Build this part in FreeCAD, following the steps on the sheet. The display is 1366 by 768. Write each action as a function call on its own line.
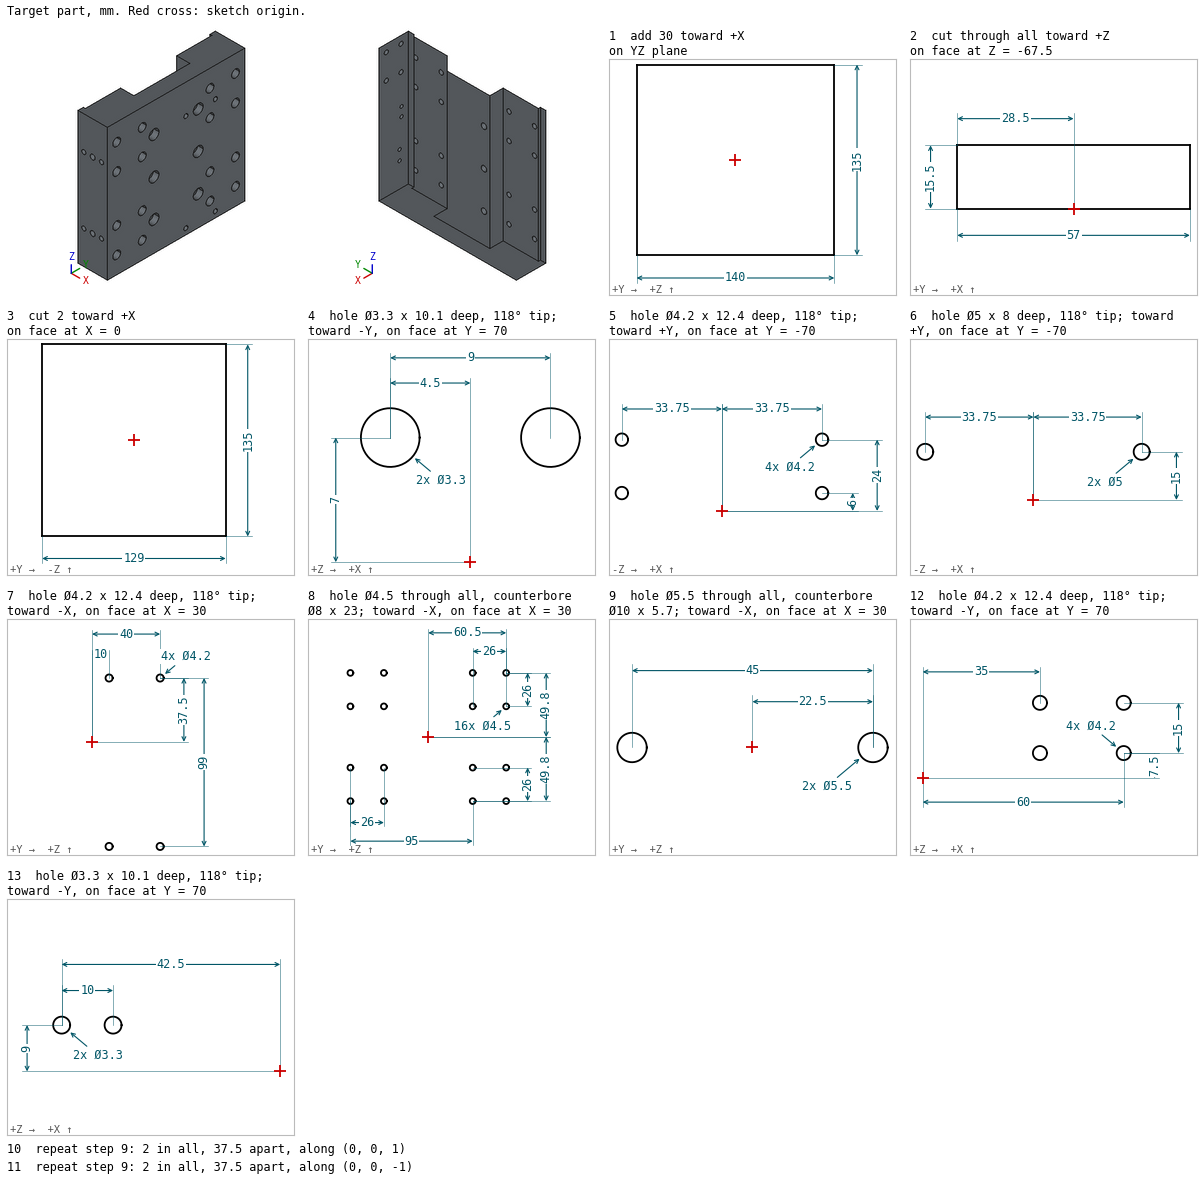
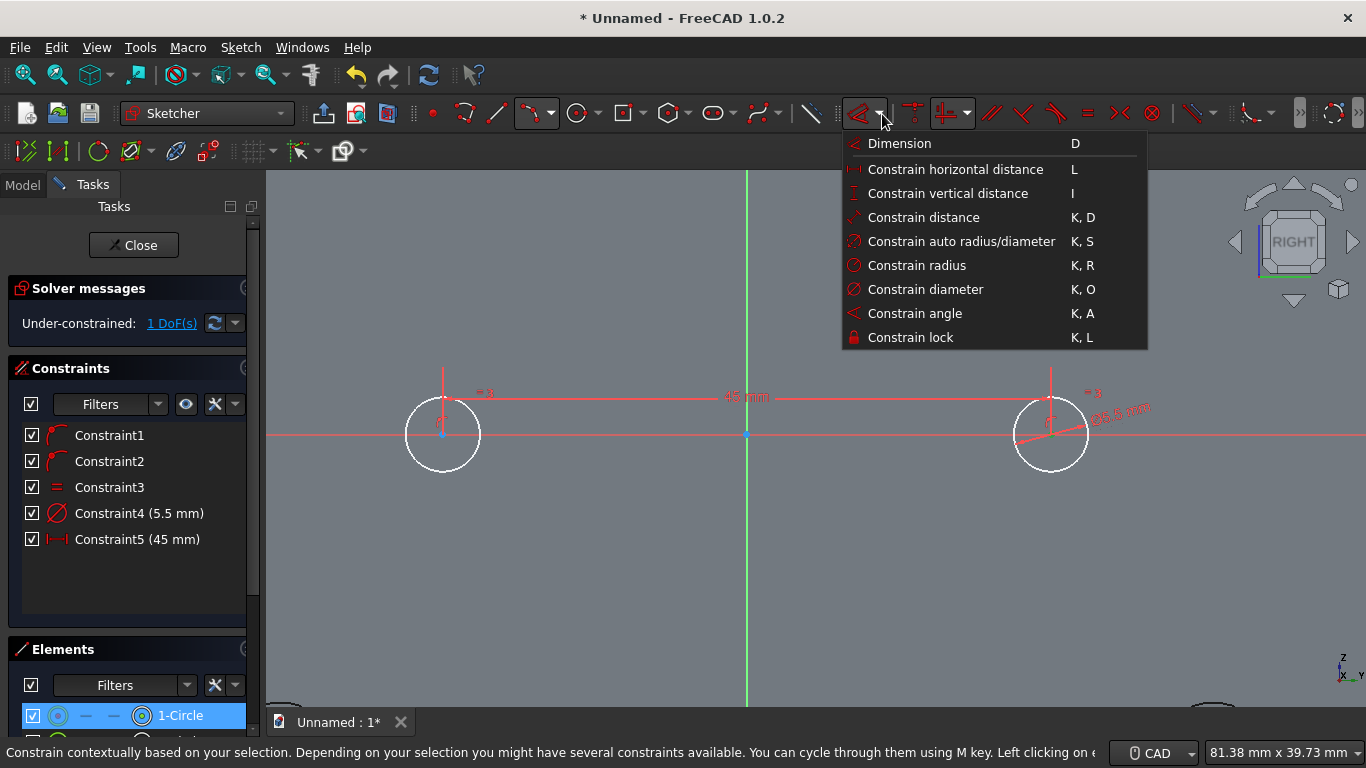
click(995, 169)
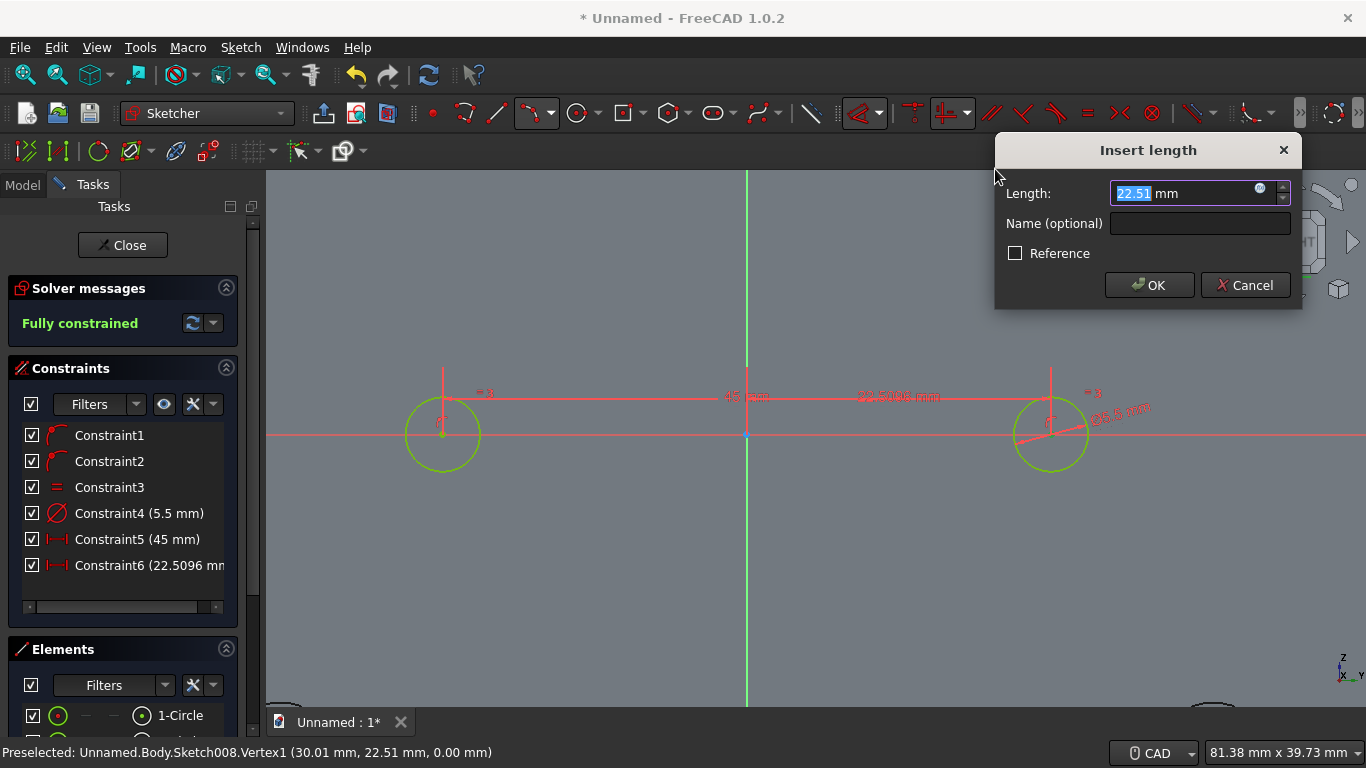
text(22.5)
key(Return)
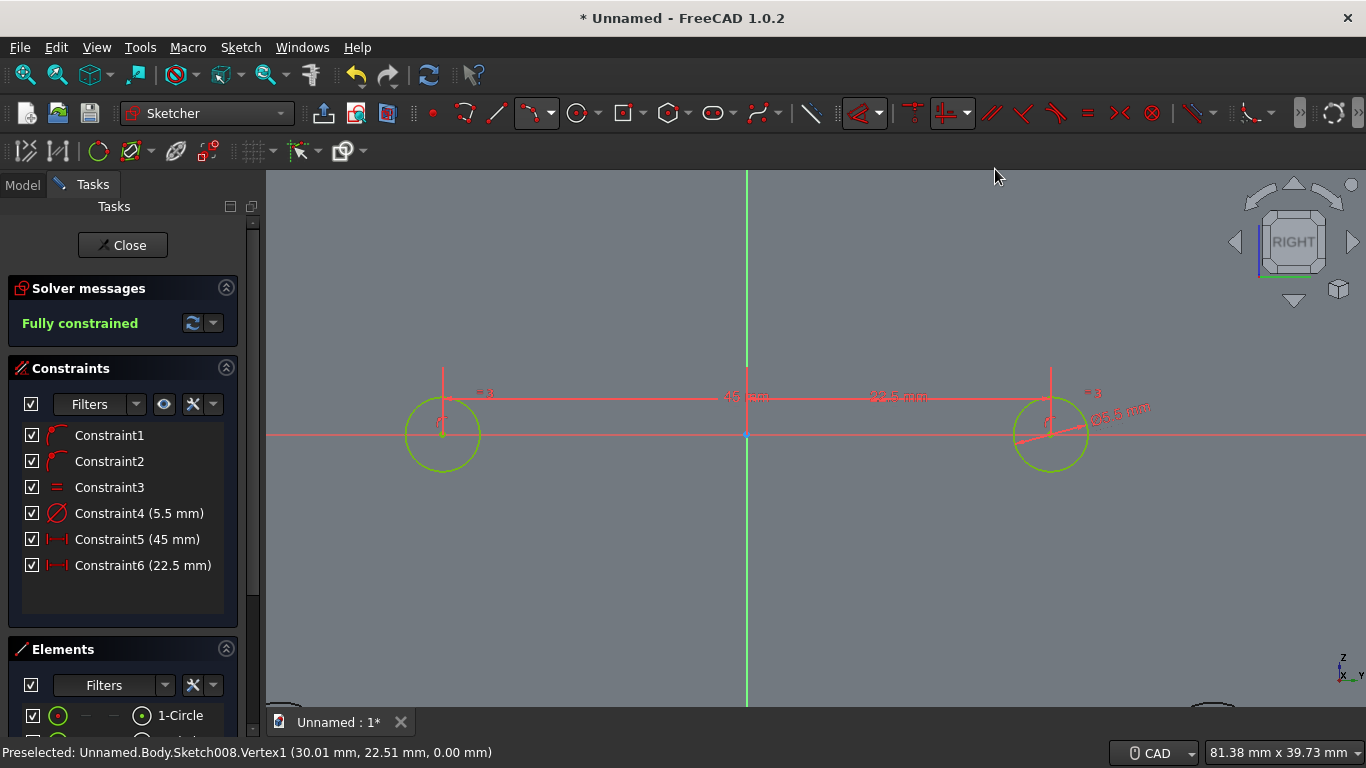
click(123, 245)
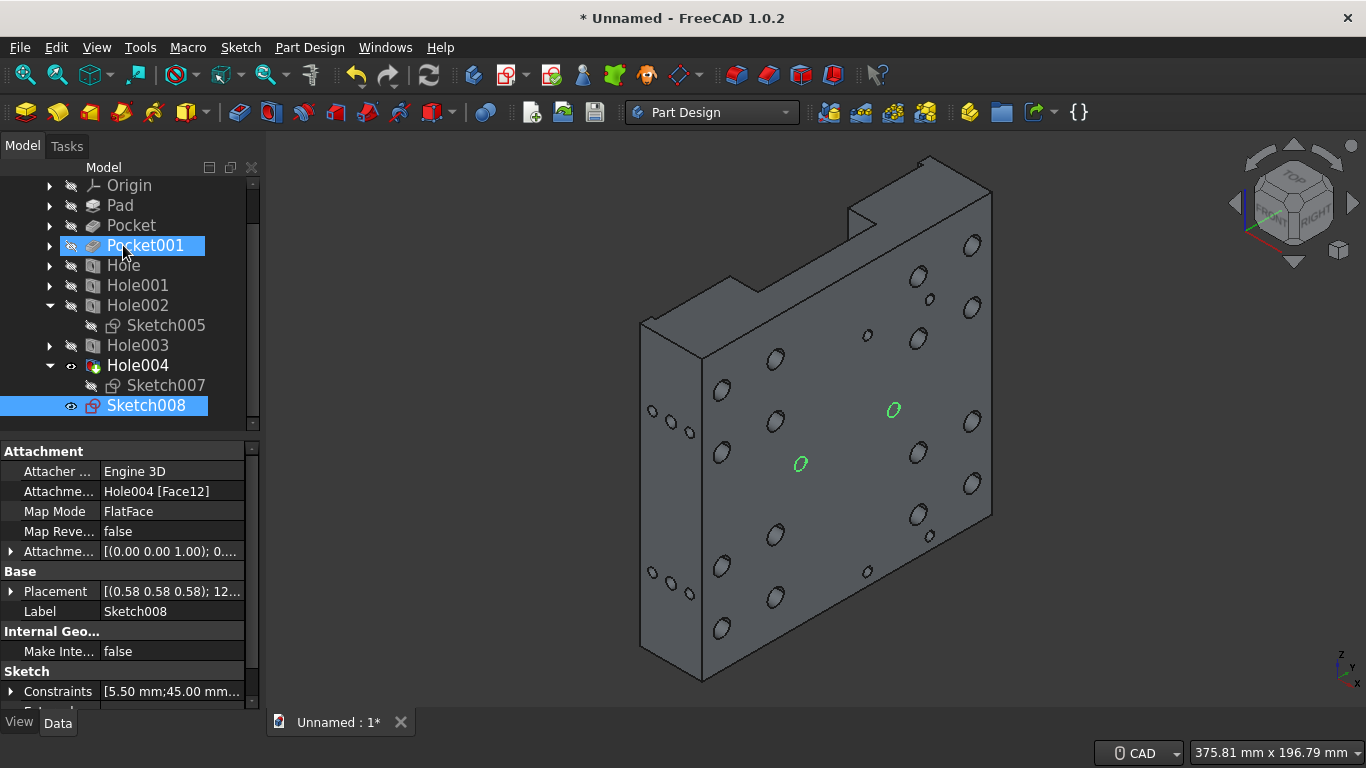
click(272, 112)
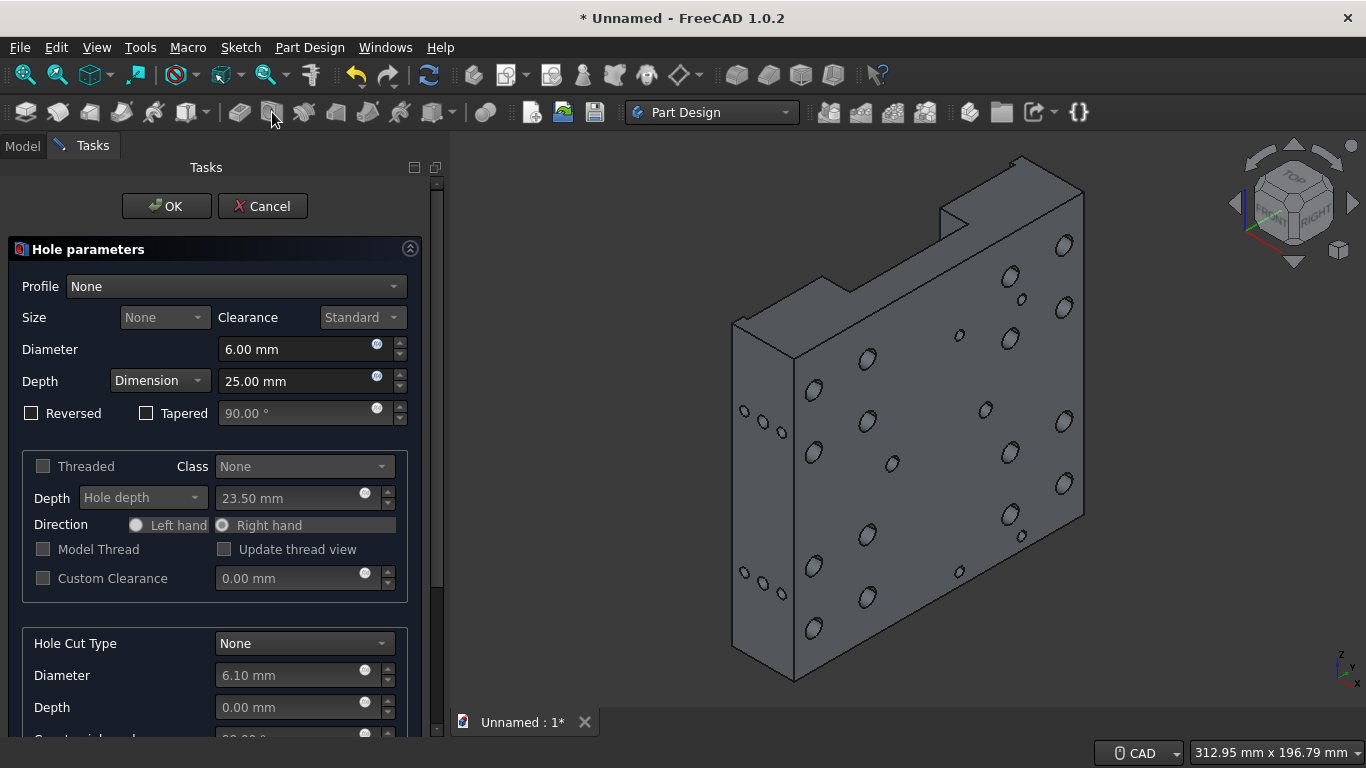
triple_click(305, 349)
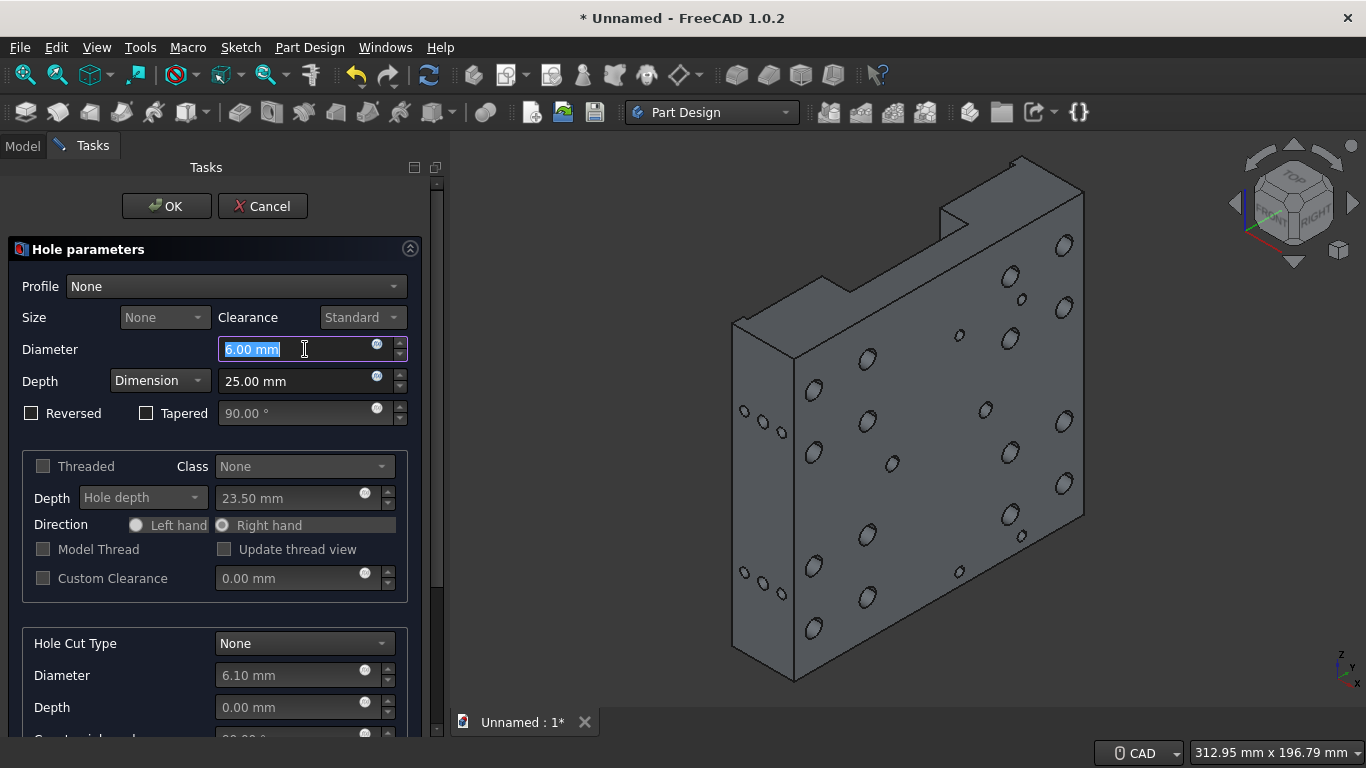
text(5.5)
key(Tab)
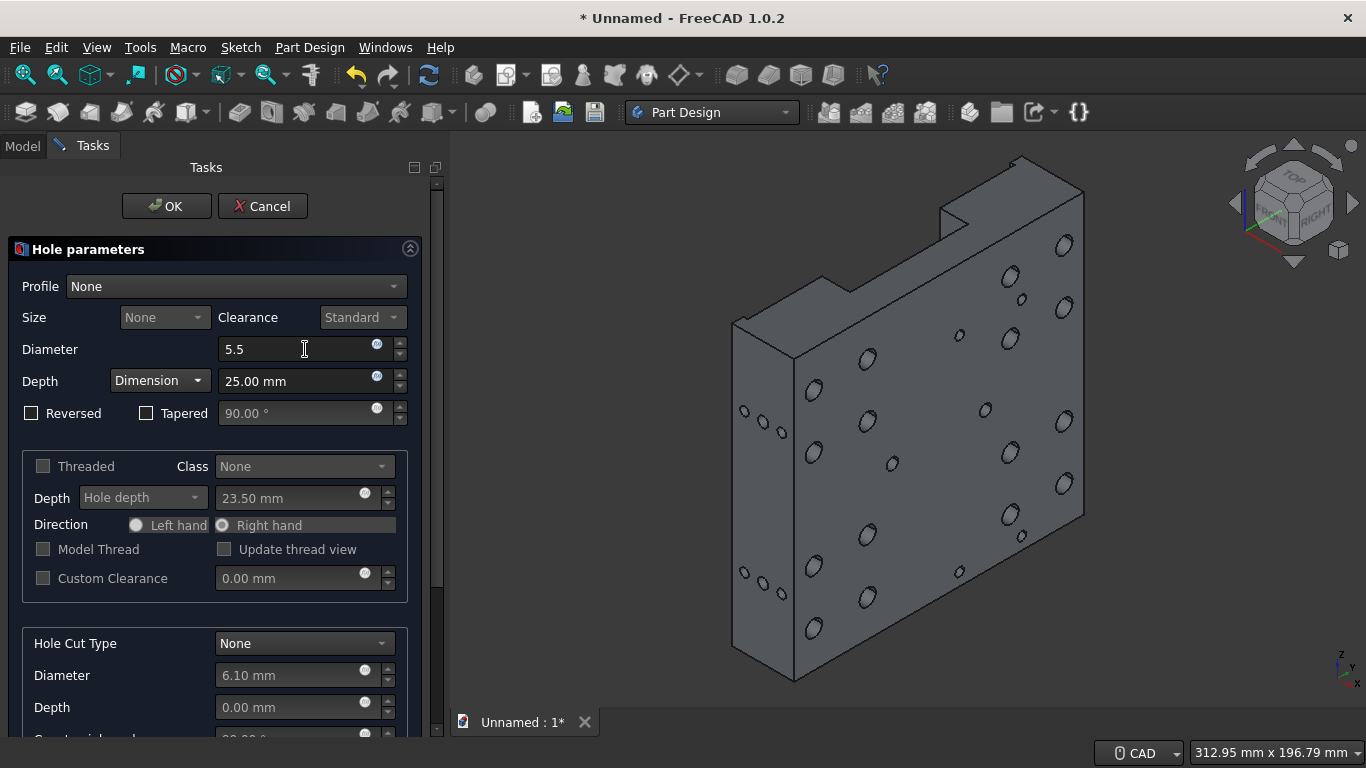
click(161, 380)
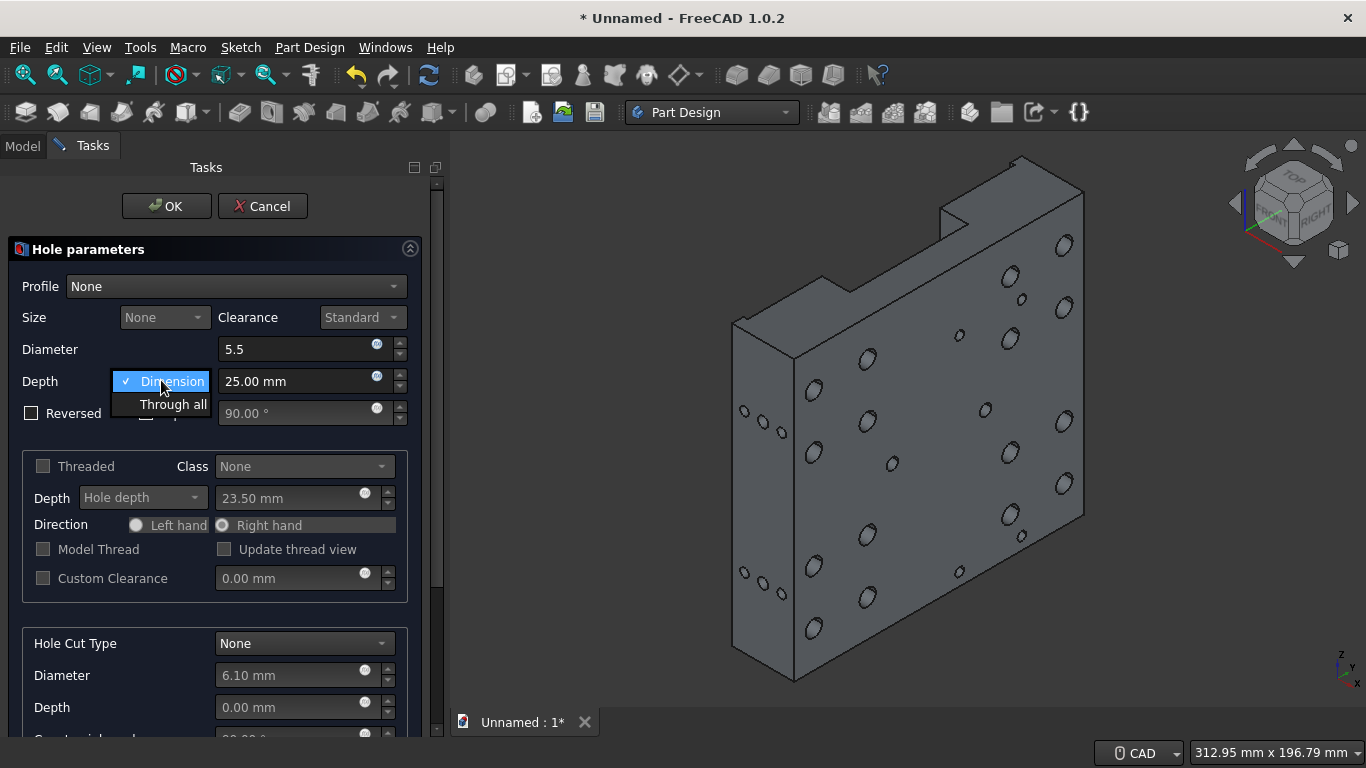
click(160, 404)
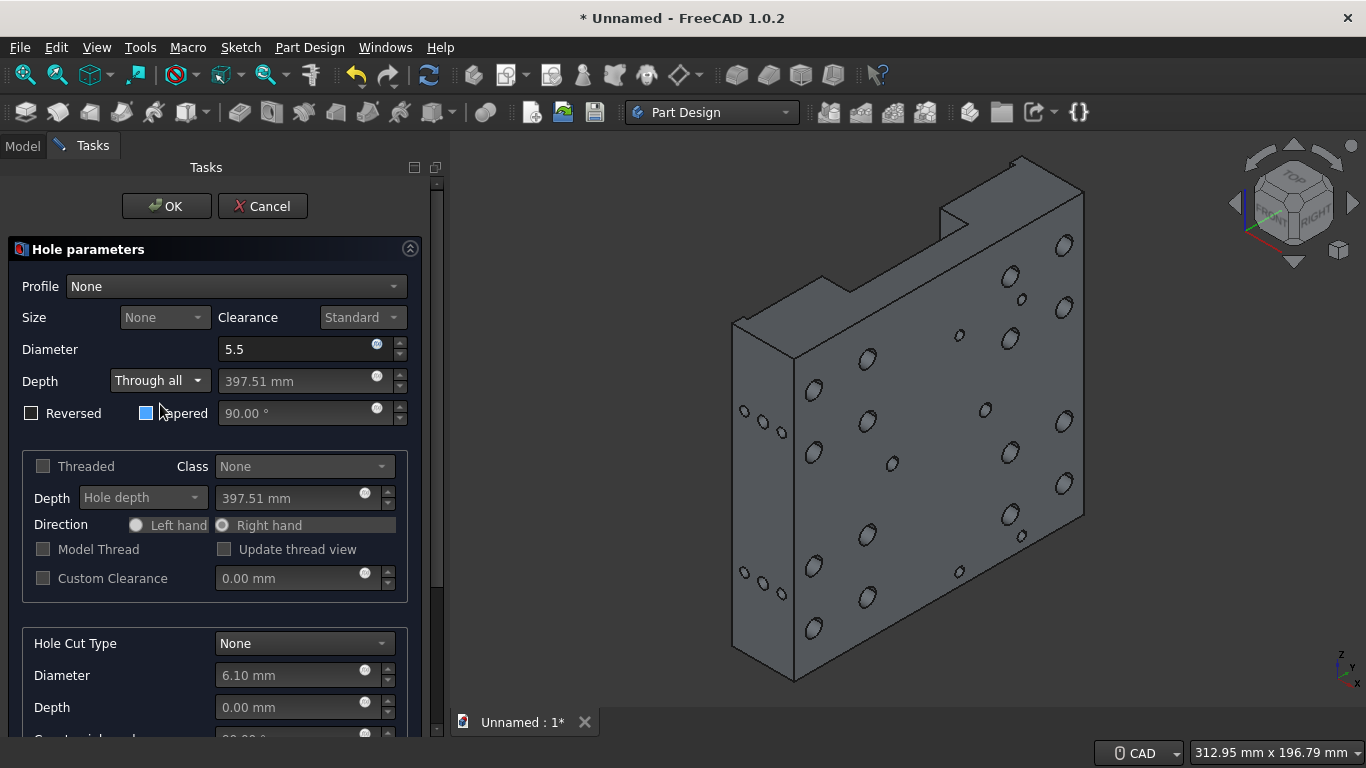
click(306, 644)